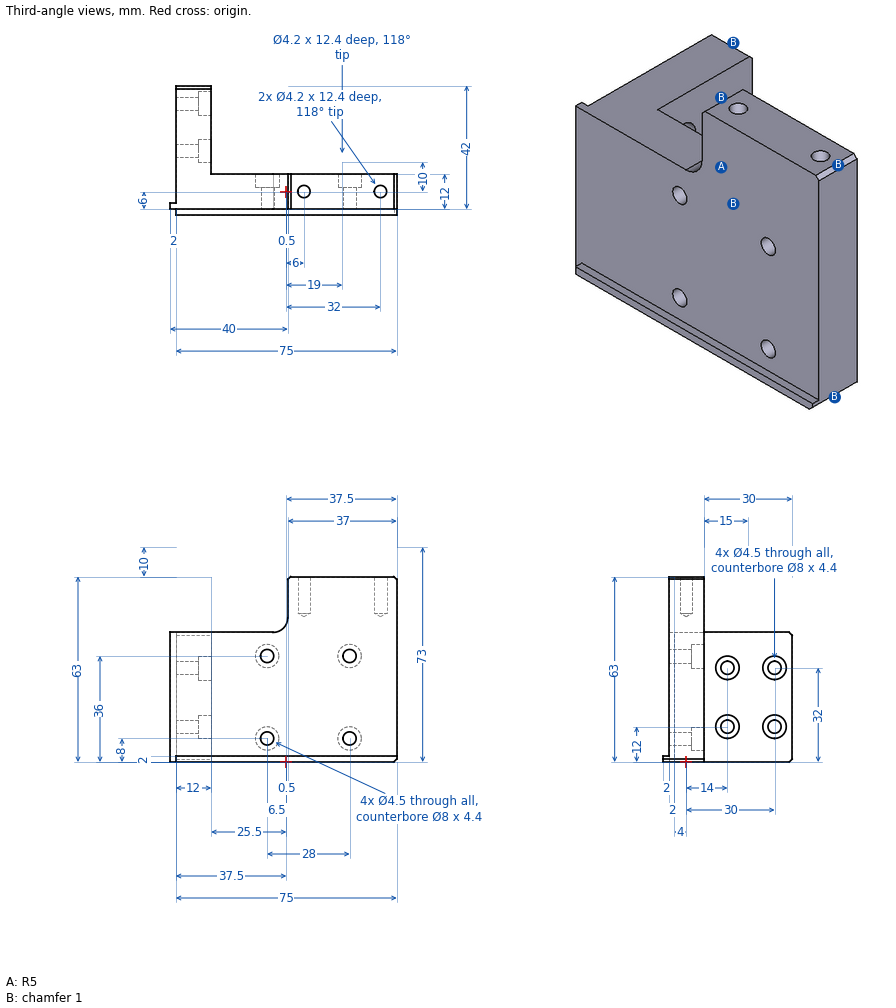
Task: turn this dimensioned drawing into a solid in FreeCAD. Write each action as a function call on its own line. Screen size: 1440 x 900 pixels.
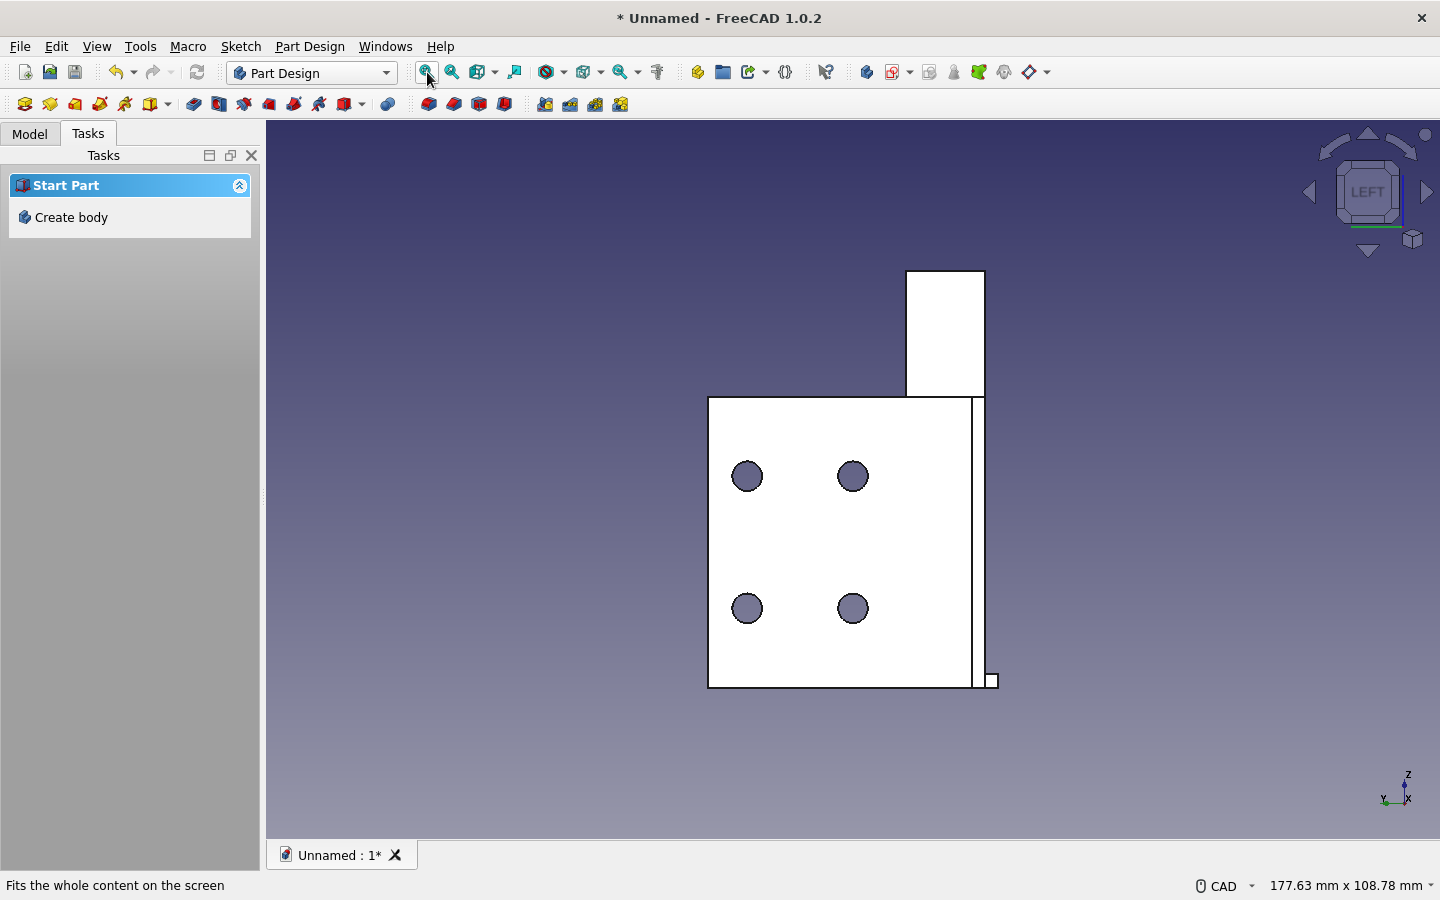
key(v)
key(3)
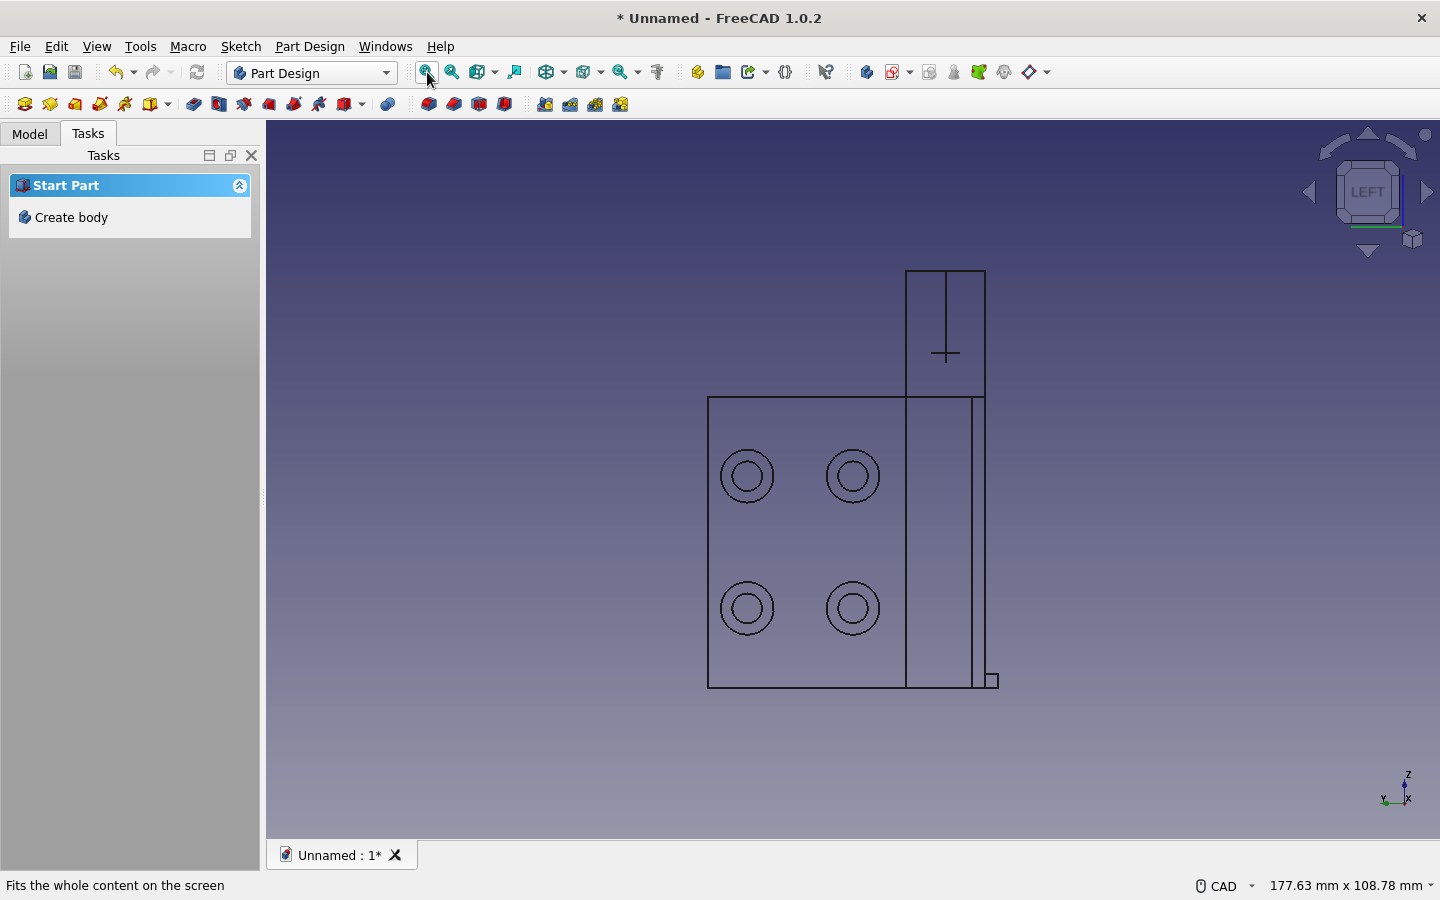
key(0)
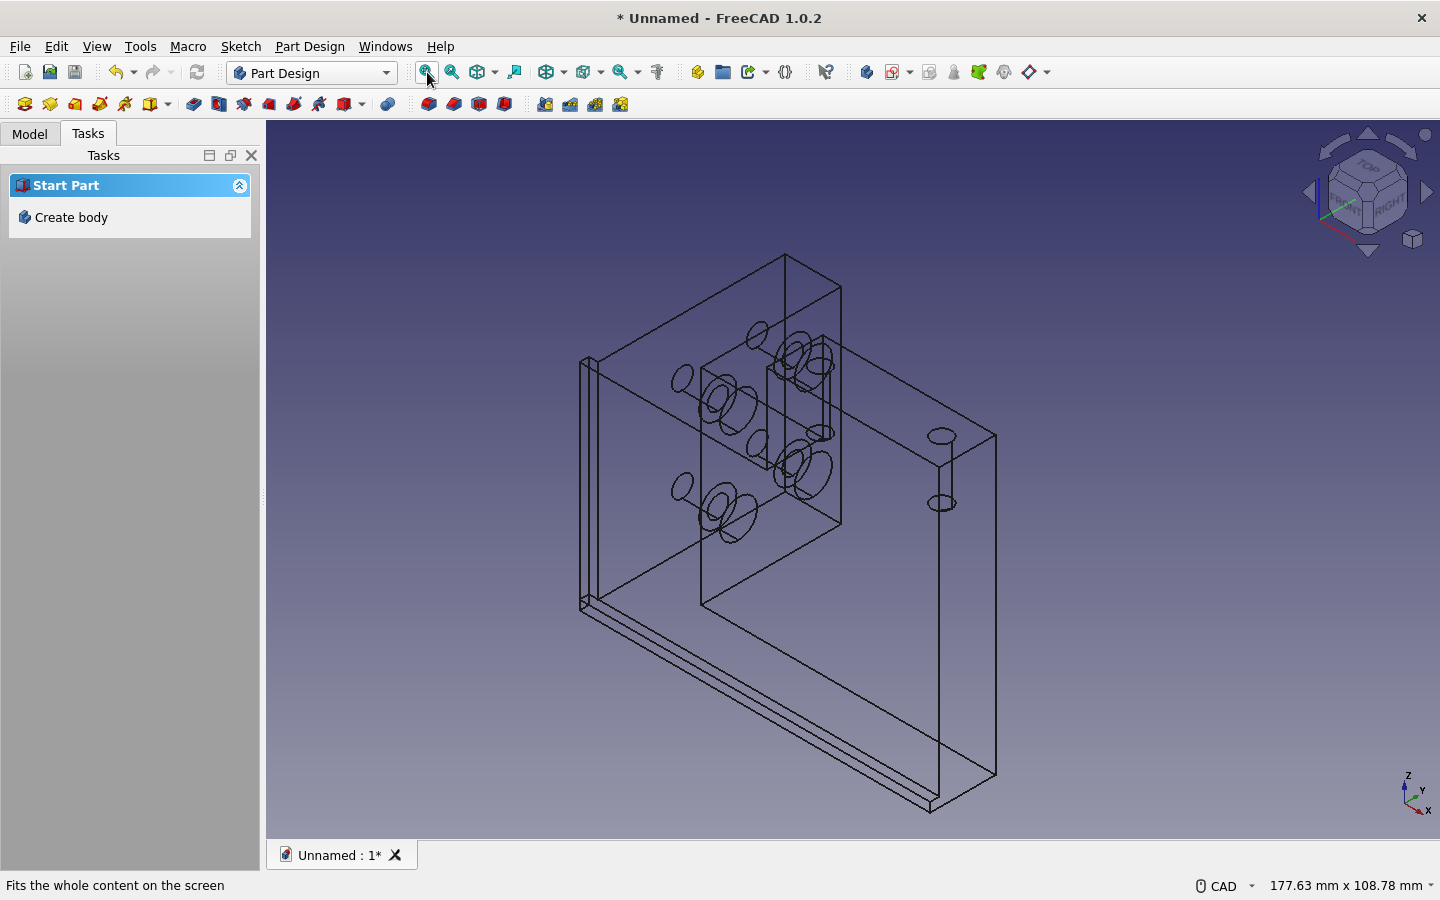
click(795, 453)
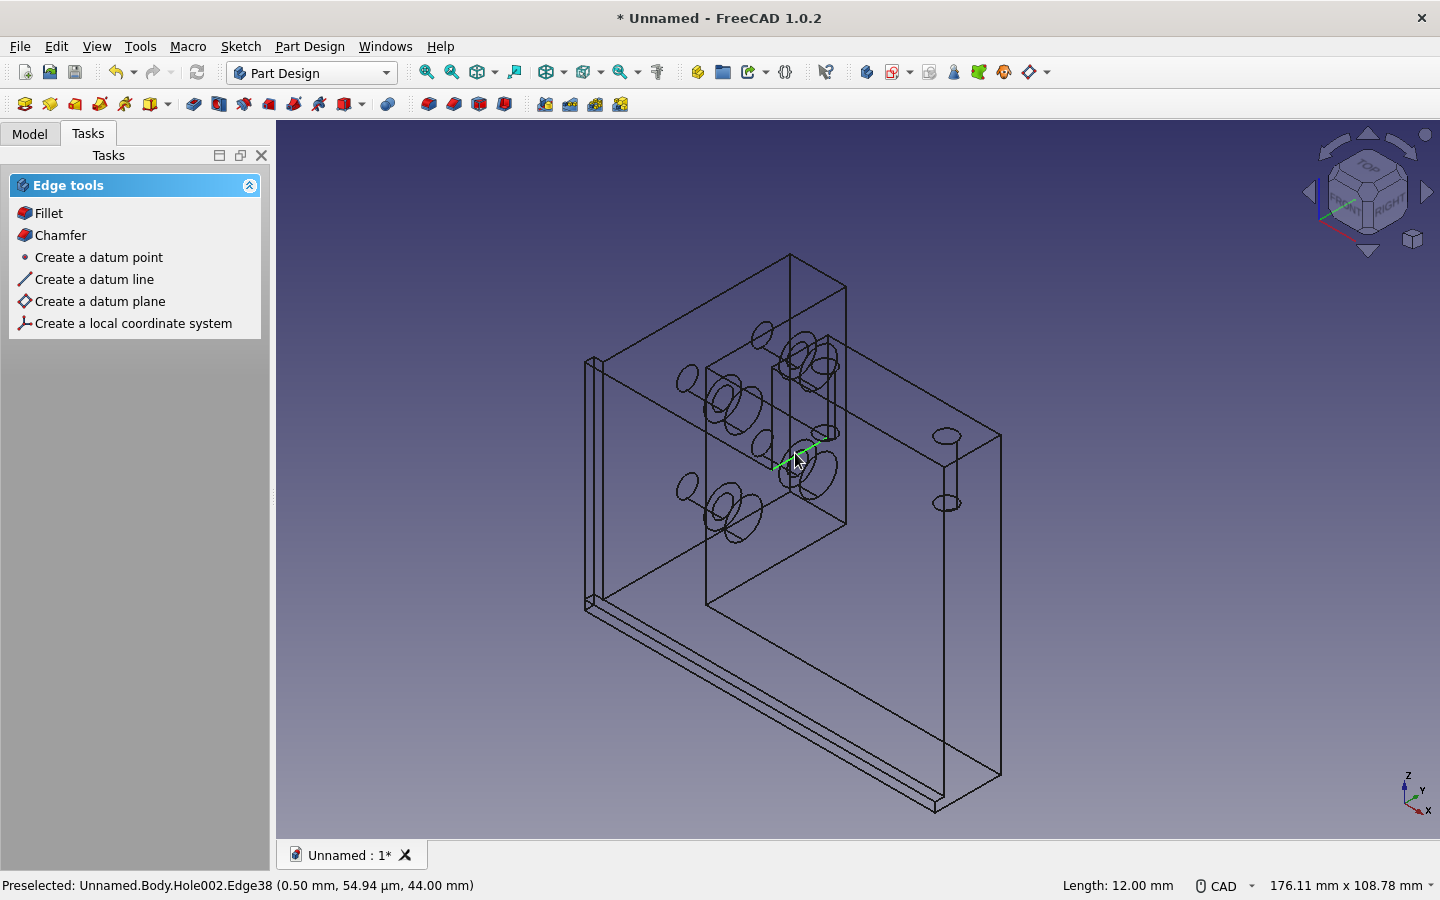
key(v)
key(1)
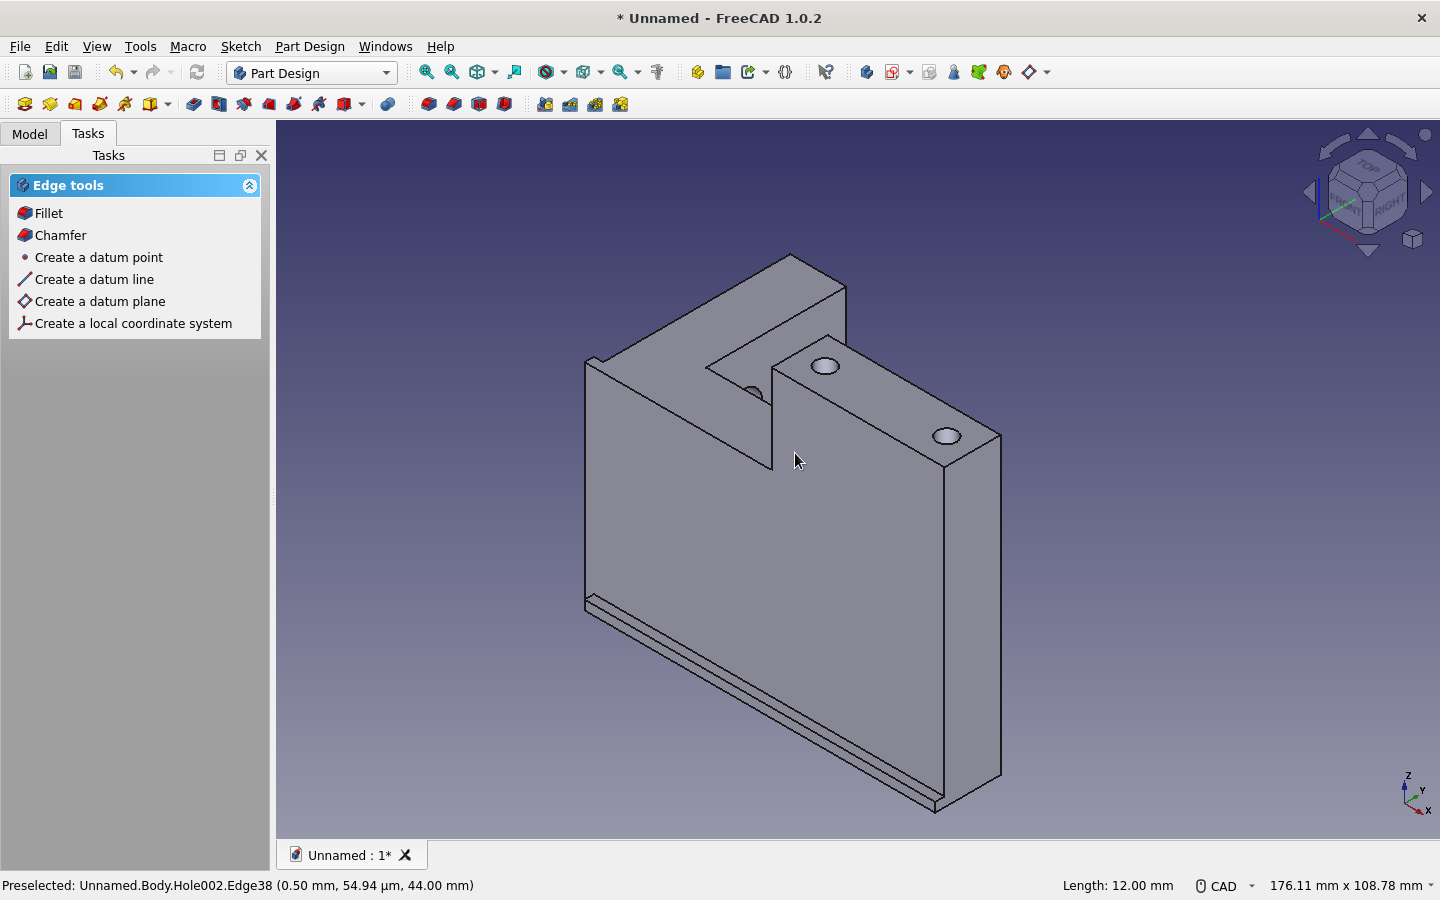
click(429, 104)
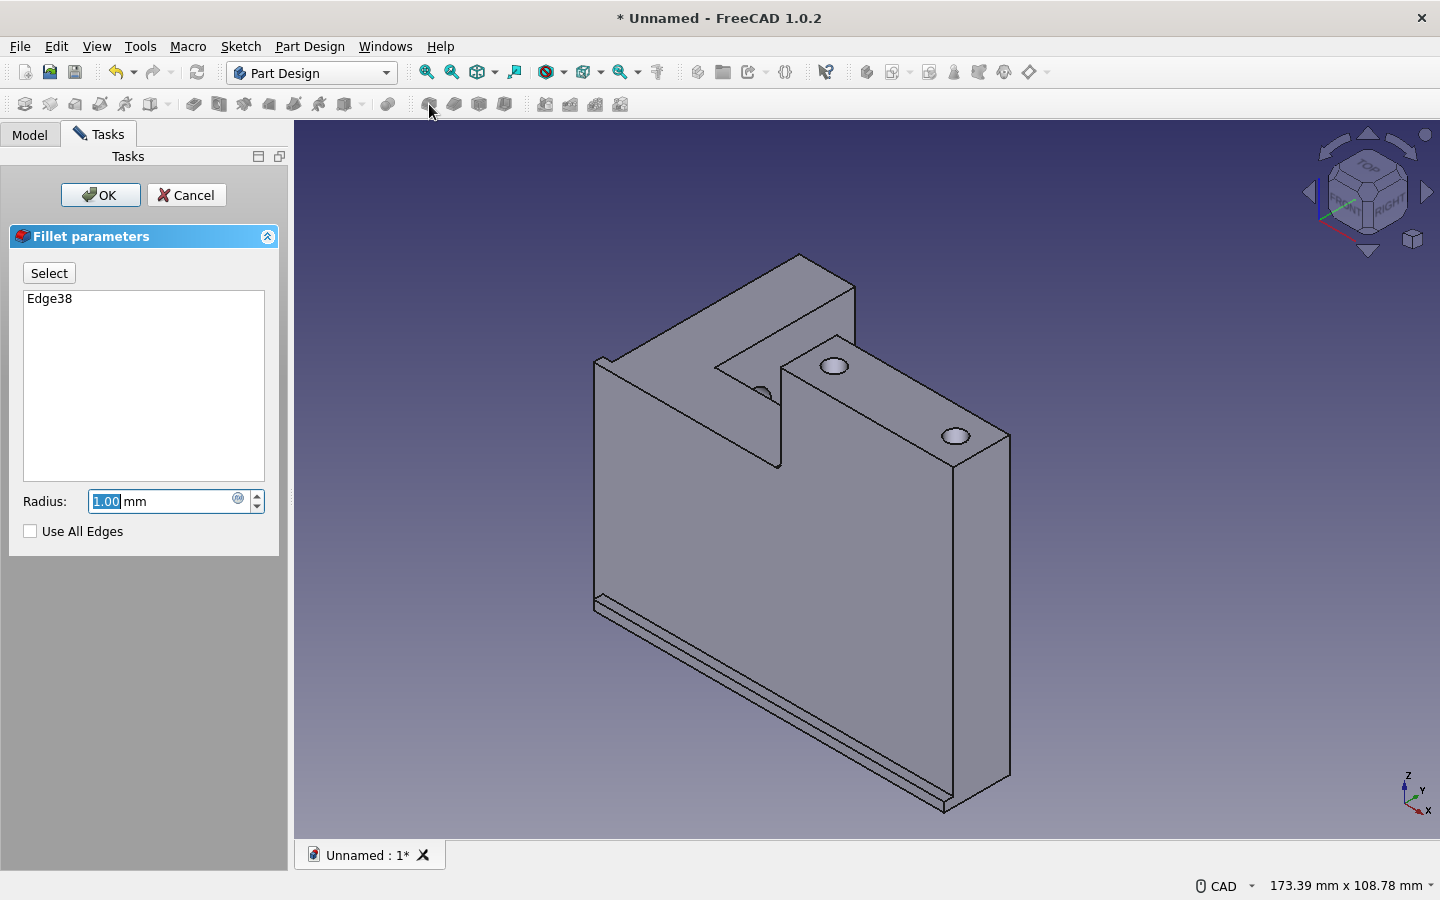
text(5)
key(Tab)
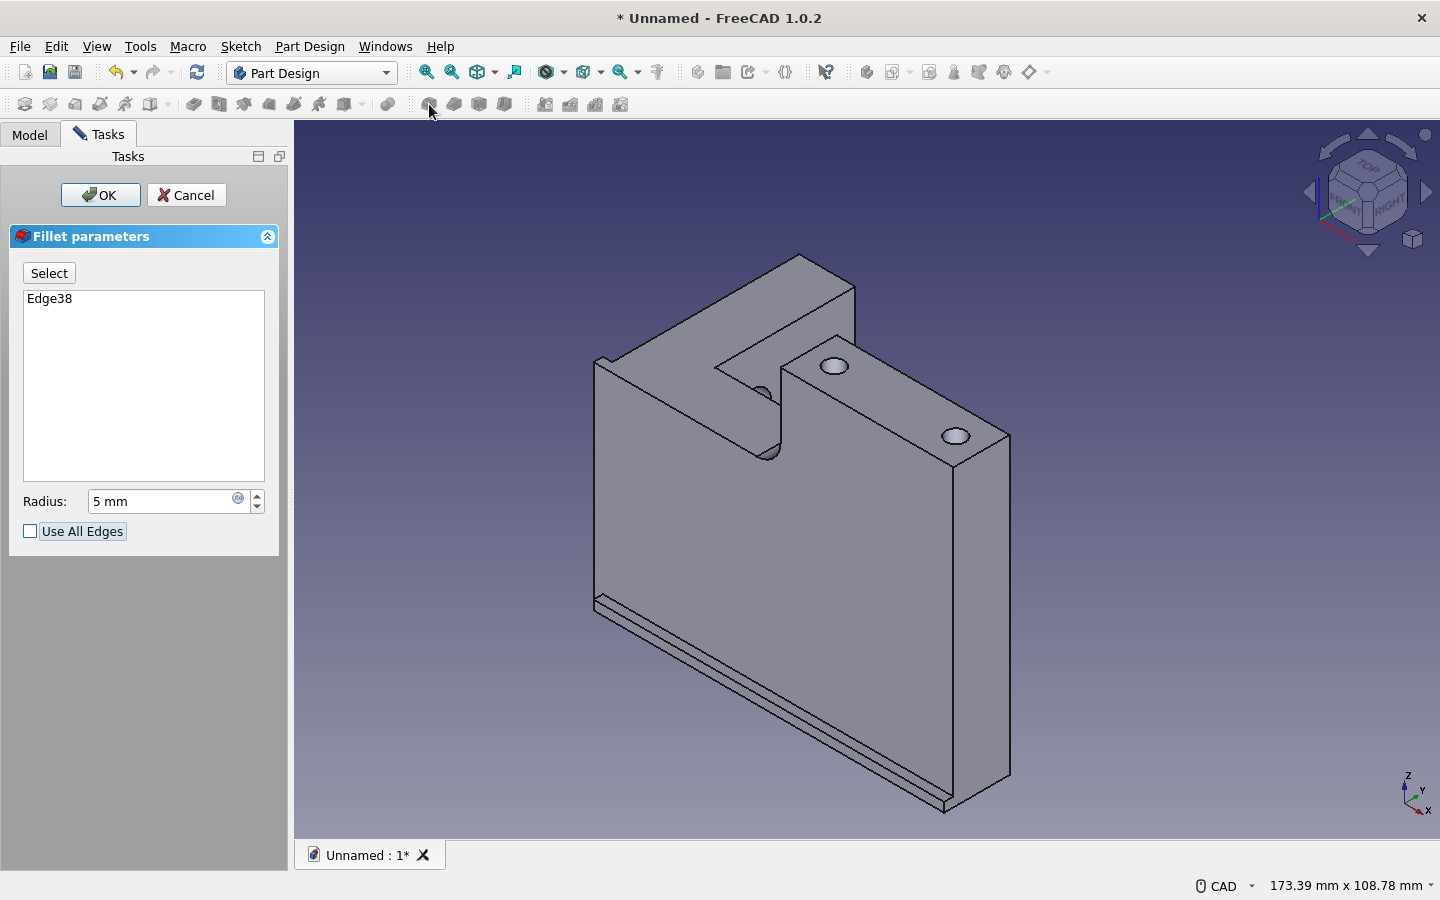
click(101, 195)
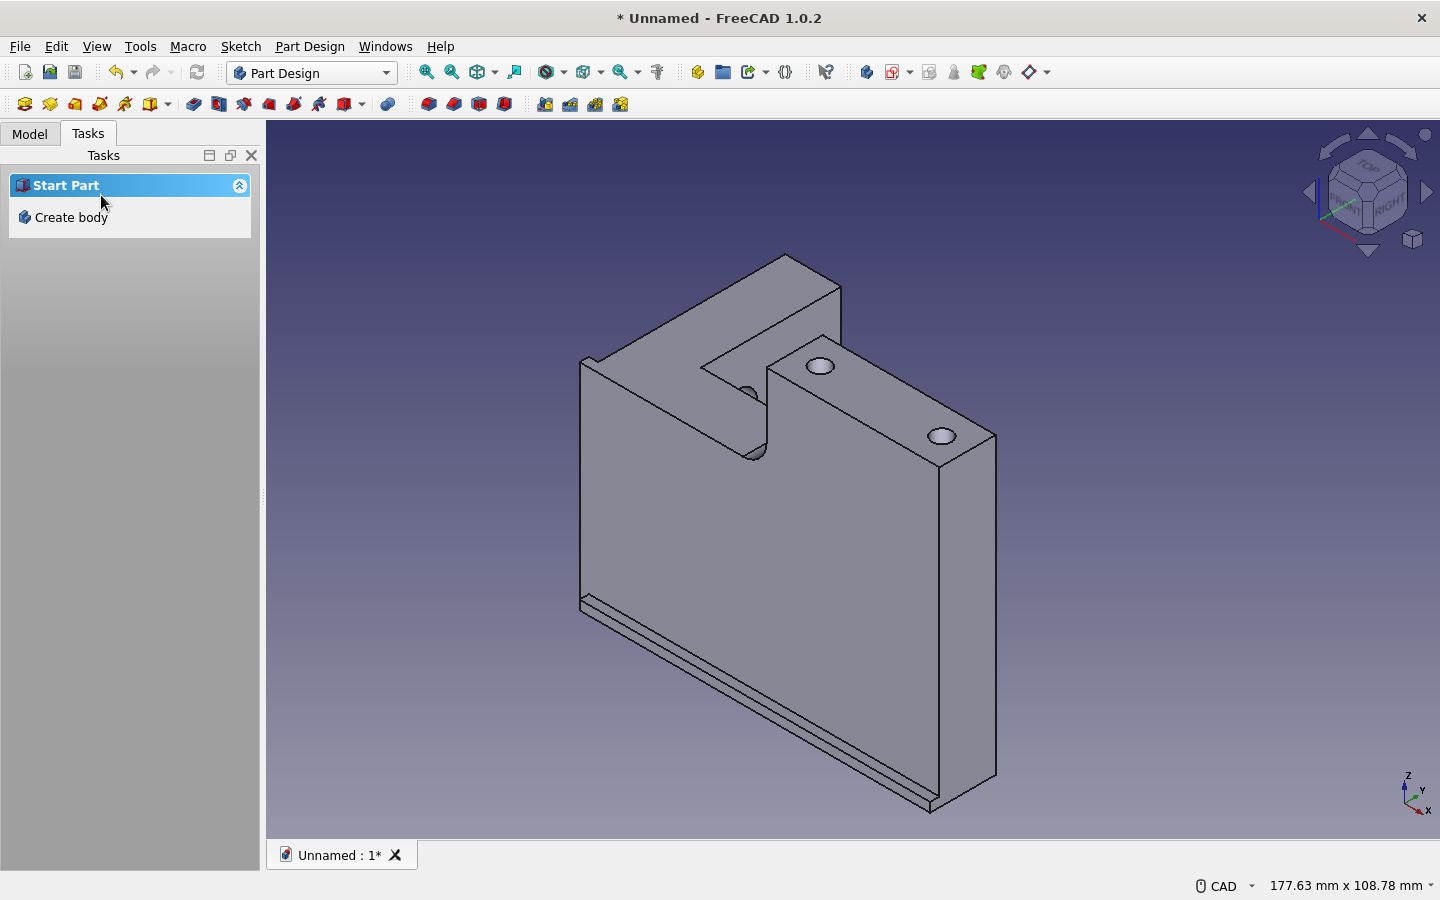
key(4)